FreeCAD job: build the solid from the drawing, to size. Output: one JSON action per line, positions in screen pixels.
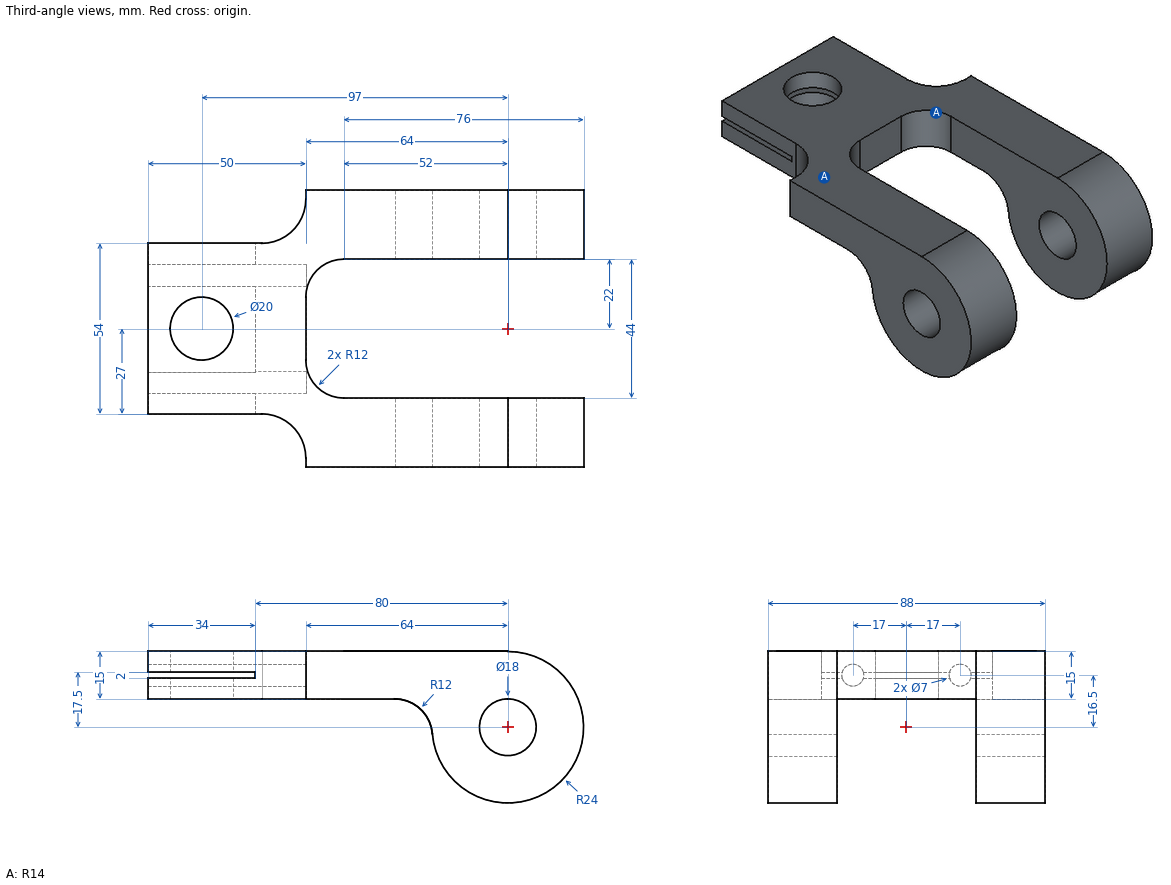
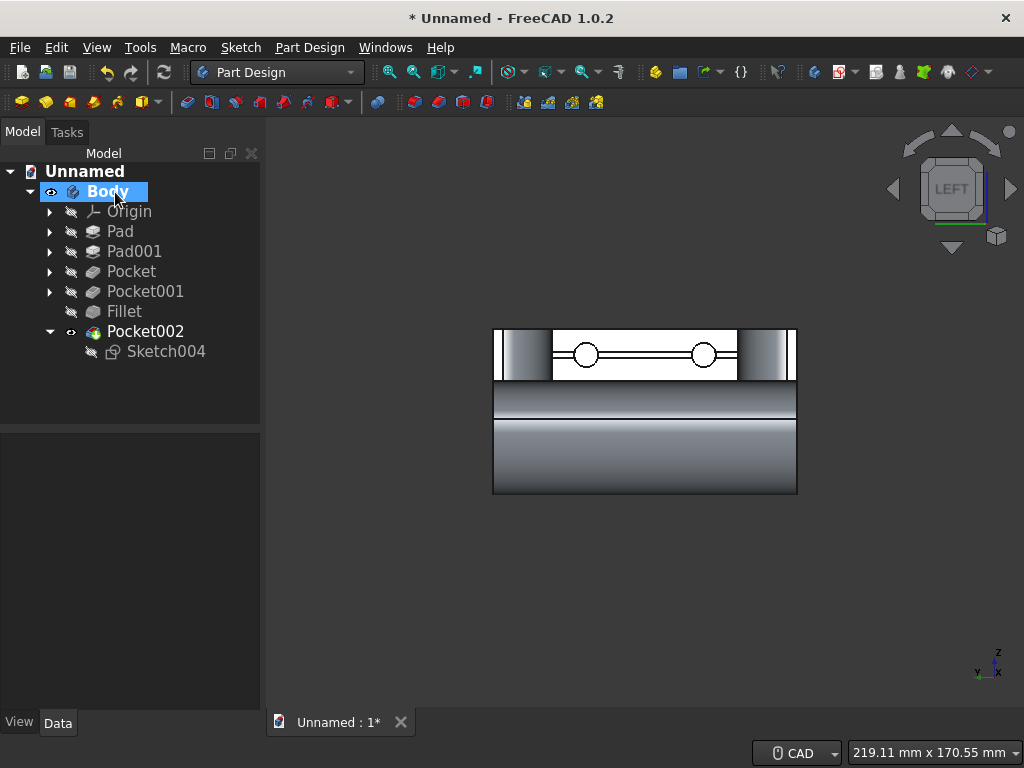
{"action": "left_click", "coordinate": [390, 72]}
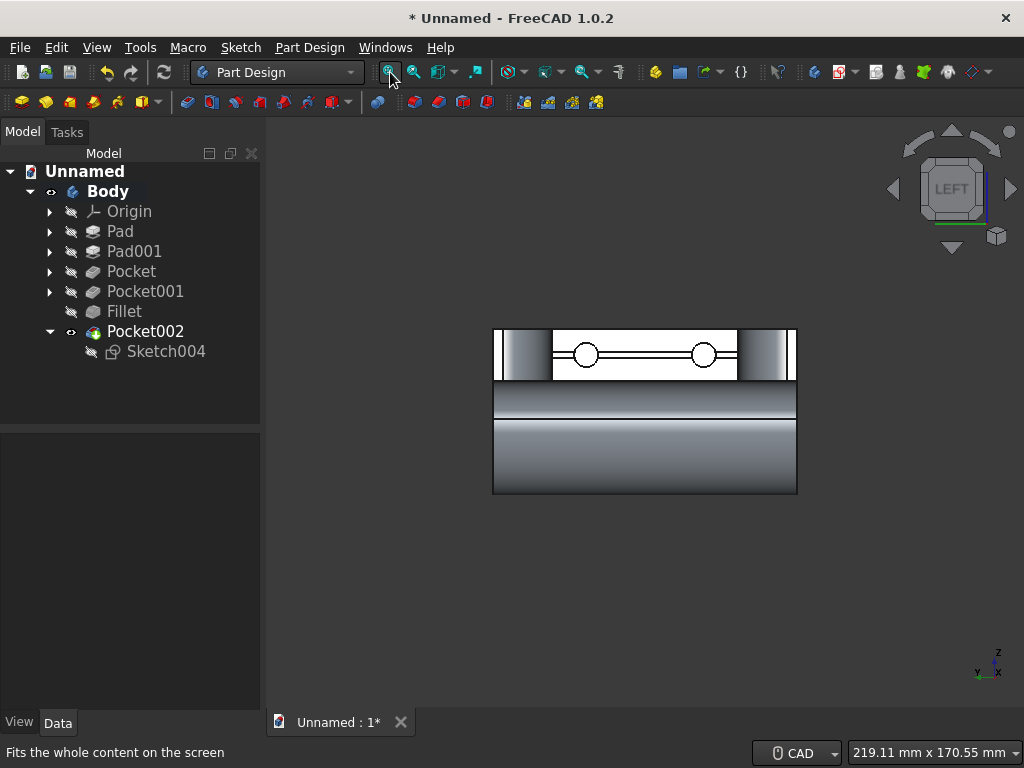
{"action": "key", "text": "5"}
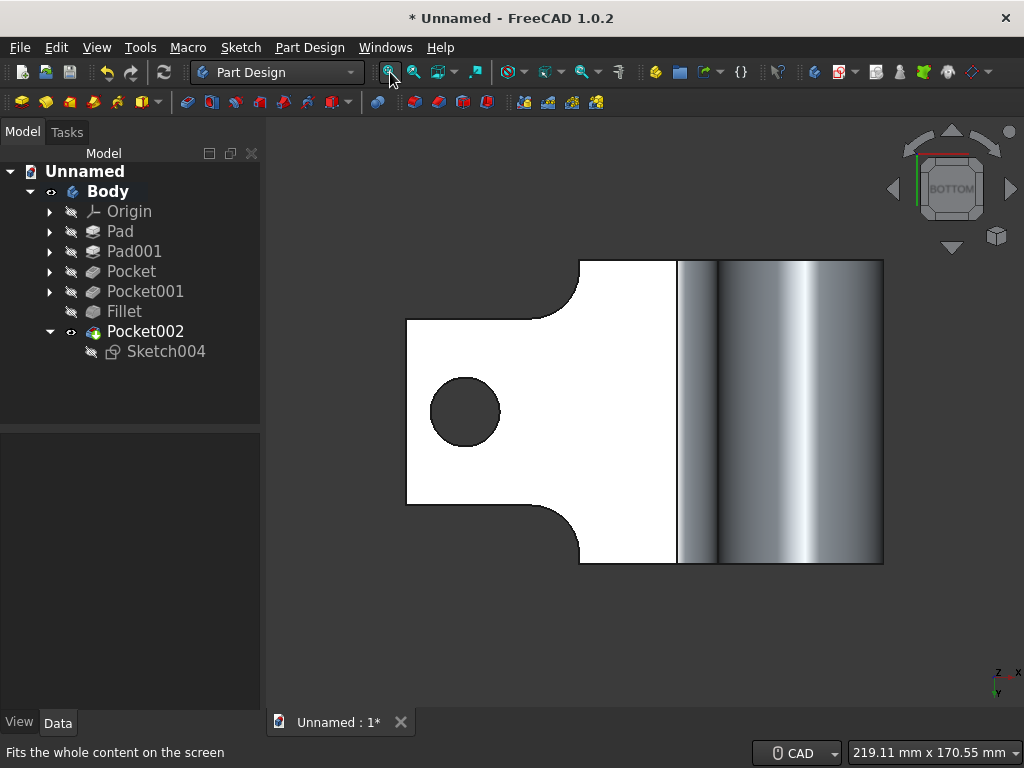
{"action": "left_click", "coordinate": [580, 411]}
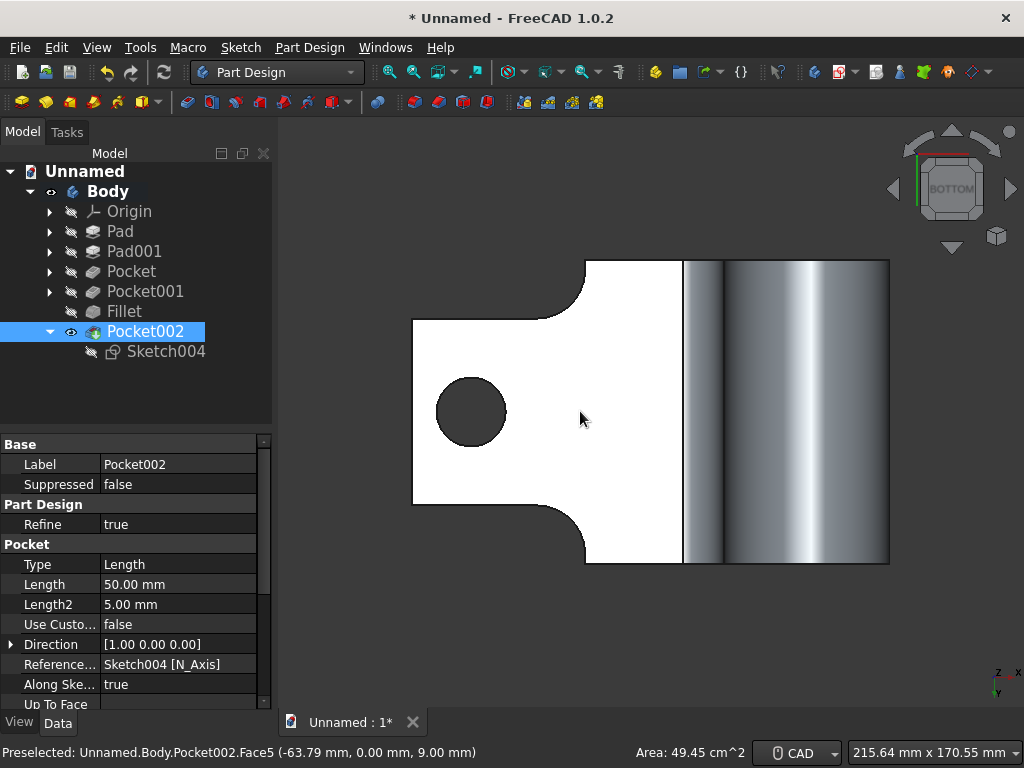
{"action": "left_click", "coordinate": [840, 72]}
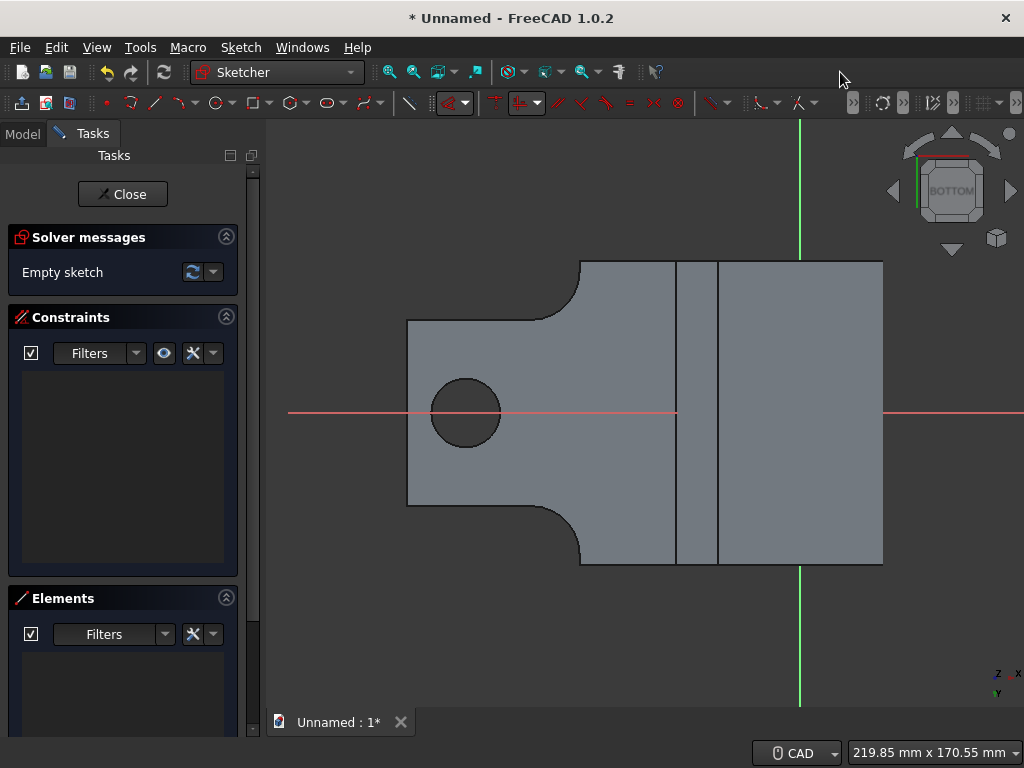
{"action": "left_click", "coordinate": [70, 104]}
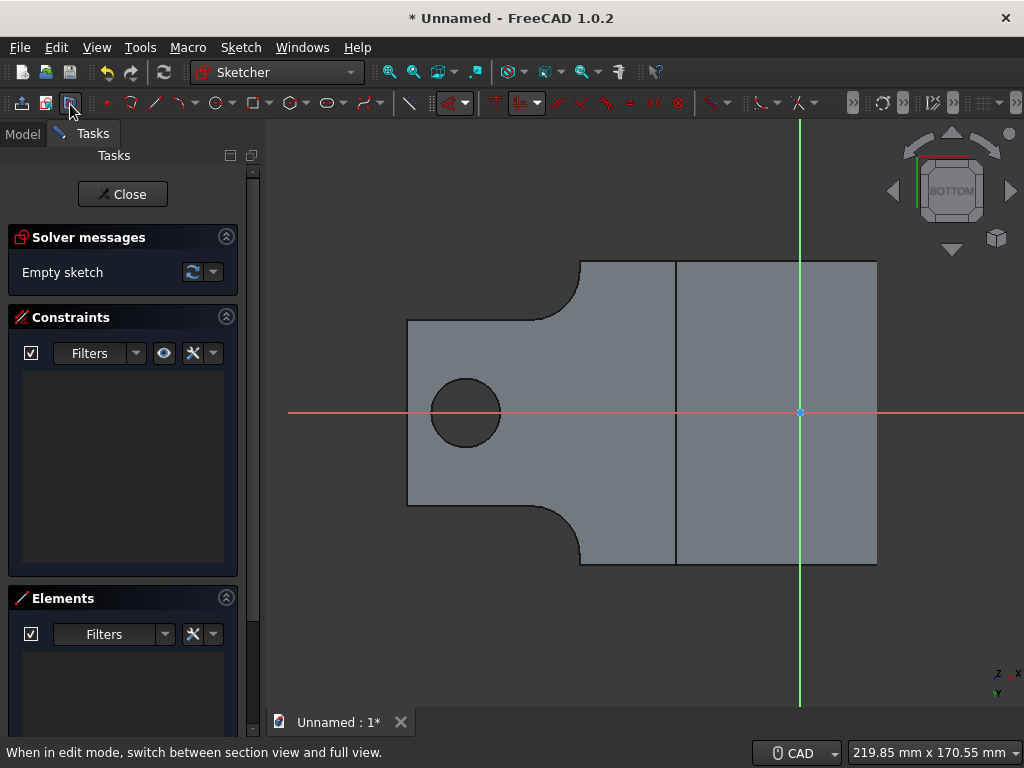
{"action": "scroll", "coordinate": [294, 413], "scroll_direction": "down", "scroll_amount": 1}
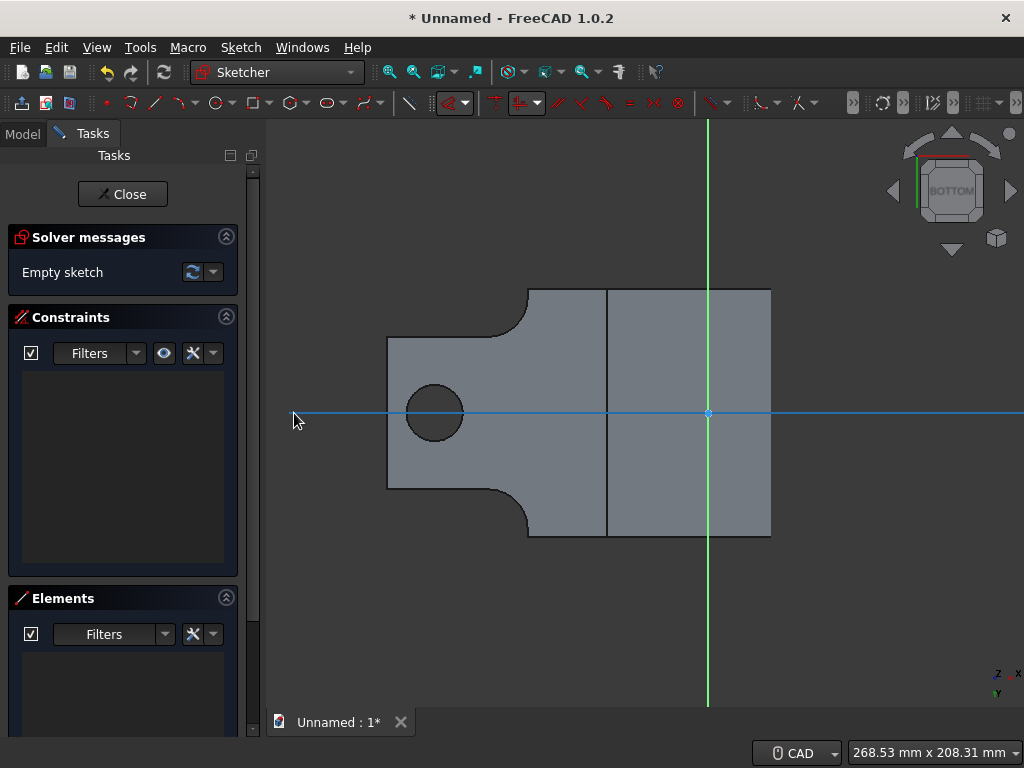
{"action": "scroll", "coordinate": [805, 413], "scroll_direction": "up", "scroll_amount": 2}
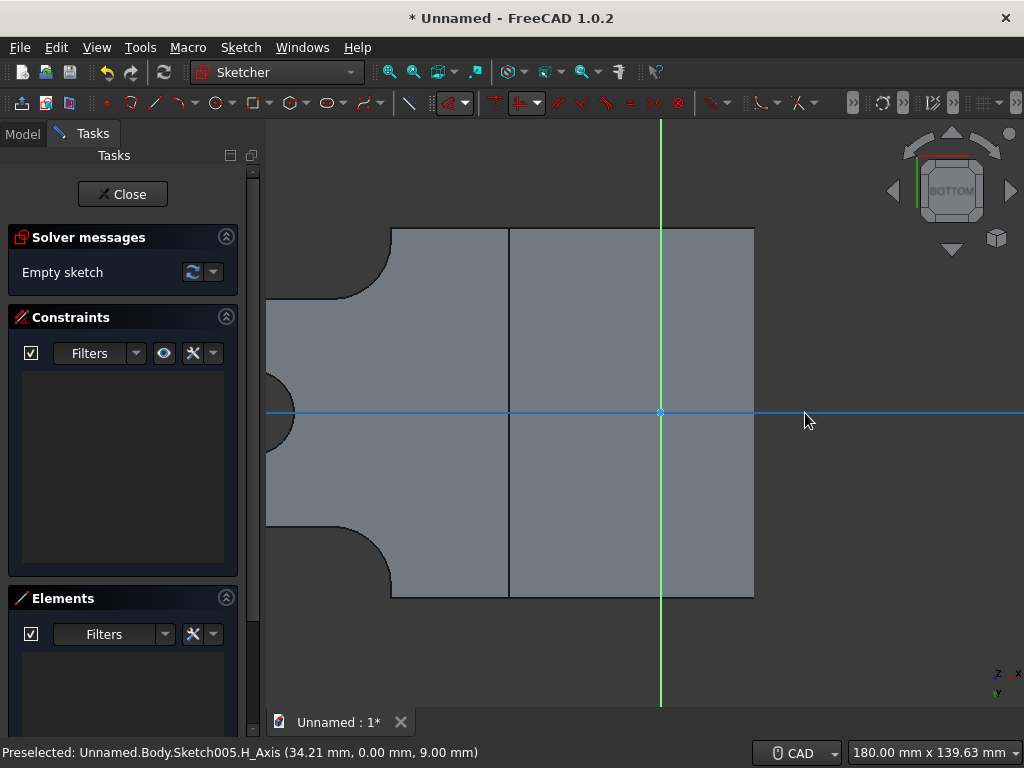
{"action": "left_click", "coordinate": [132, 104]}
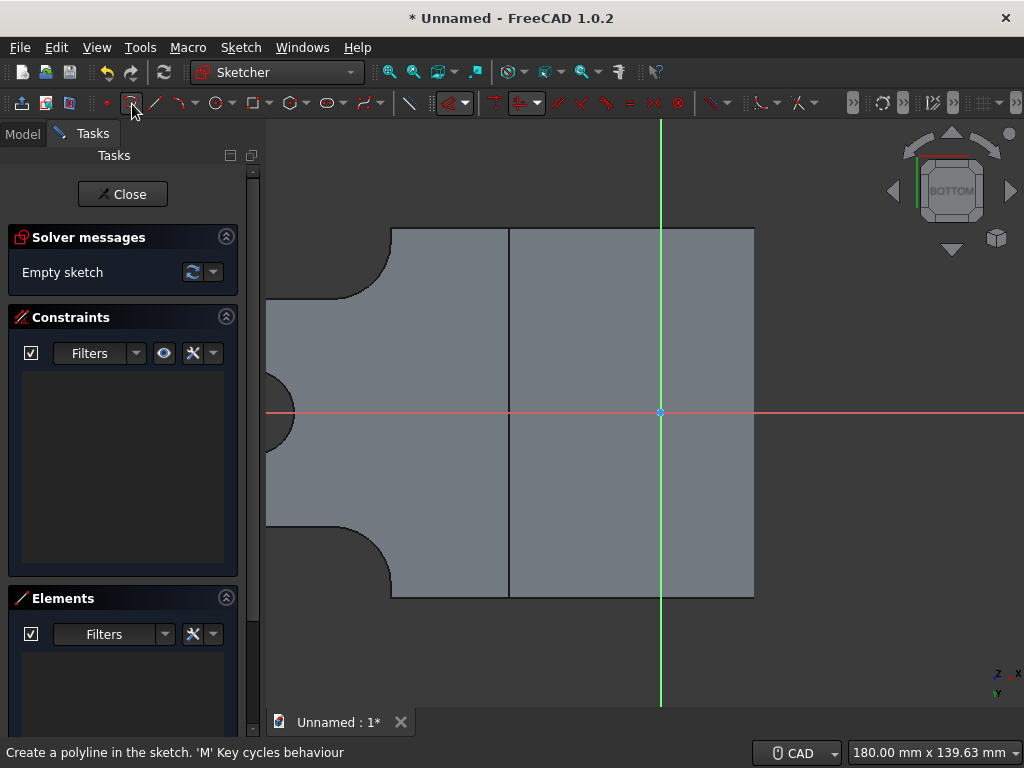
{"action": "left_click", "coordinate": [442, 506]}
{"action": "left_click", "coordinate": [762, 506]}
{"action": "left_click", "coordinate": [762, 320]}
{"action": "left_click", "coordinate": [442, 320]}
{"action": "right_click", "coordinate": [442, 320]}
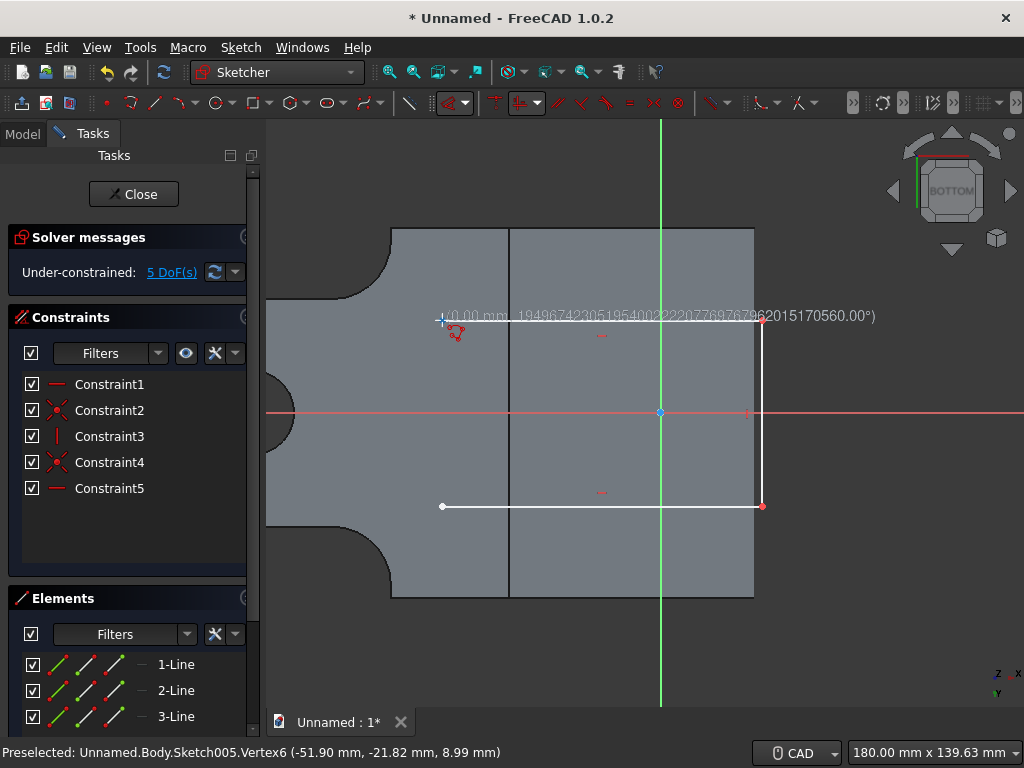
{"action": "left_click", "coordinate": [156, 104]}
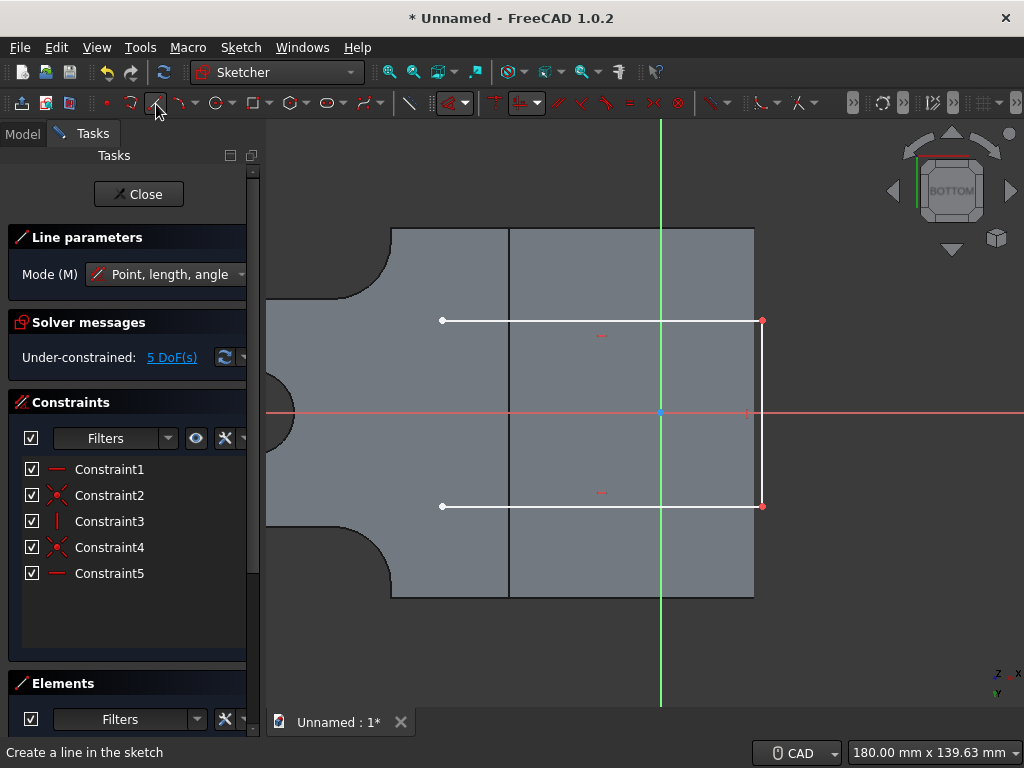
{"action": "left_click", "coordinate": [391, 371]}
{"action": "left_click", "coordinate": [391, 455]}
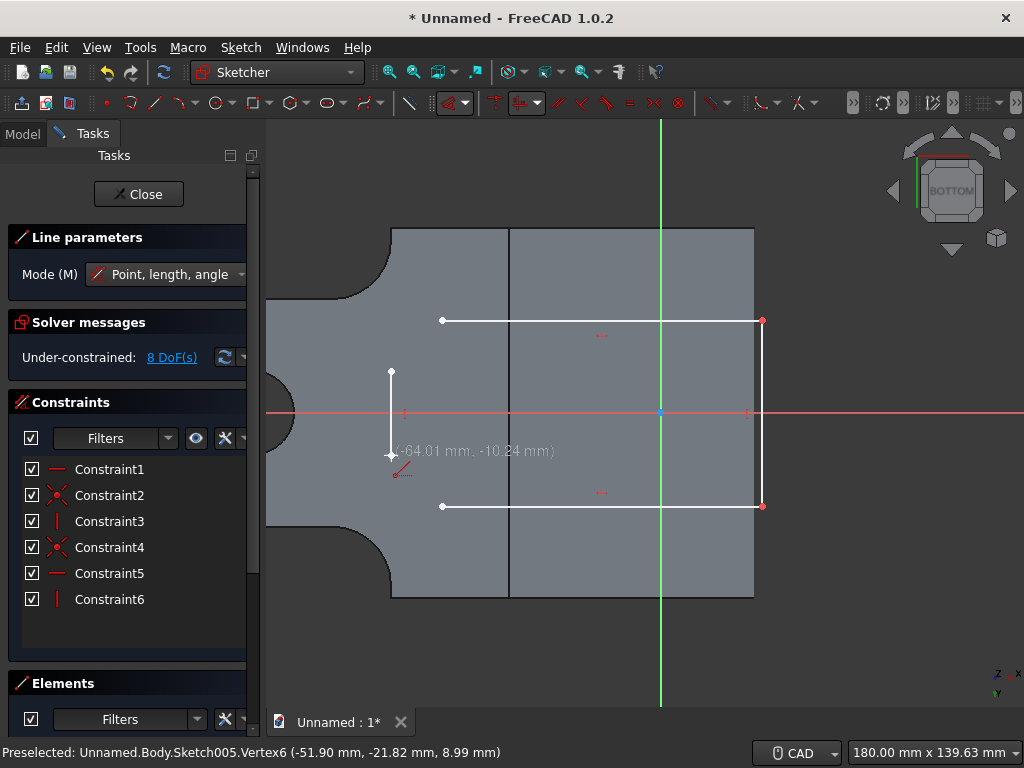
{"action": "left_click", "coordinate": [180, 104]}